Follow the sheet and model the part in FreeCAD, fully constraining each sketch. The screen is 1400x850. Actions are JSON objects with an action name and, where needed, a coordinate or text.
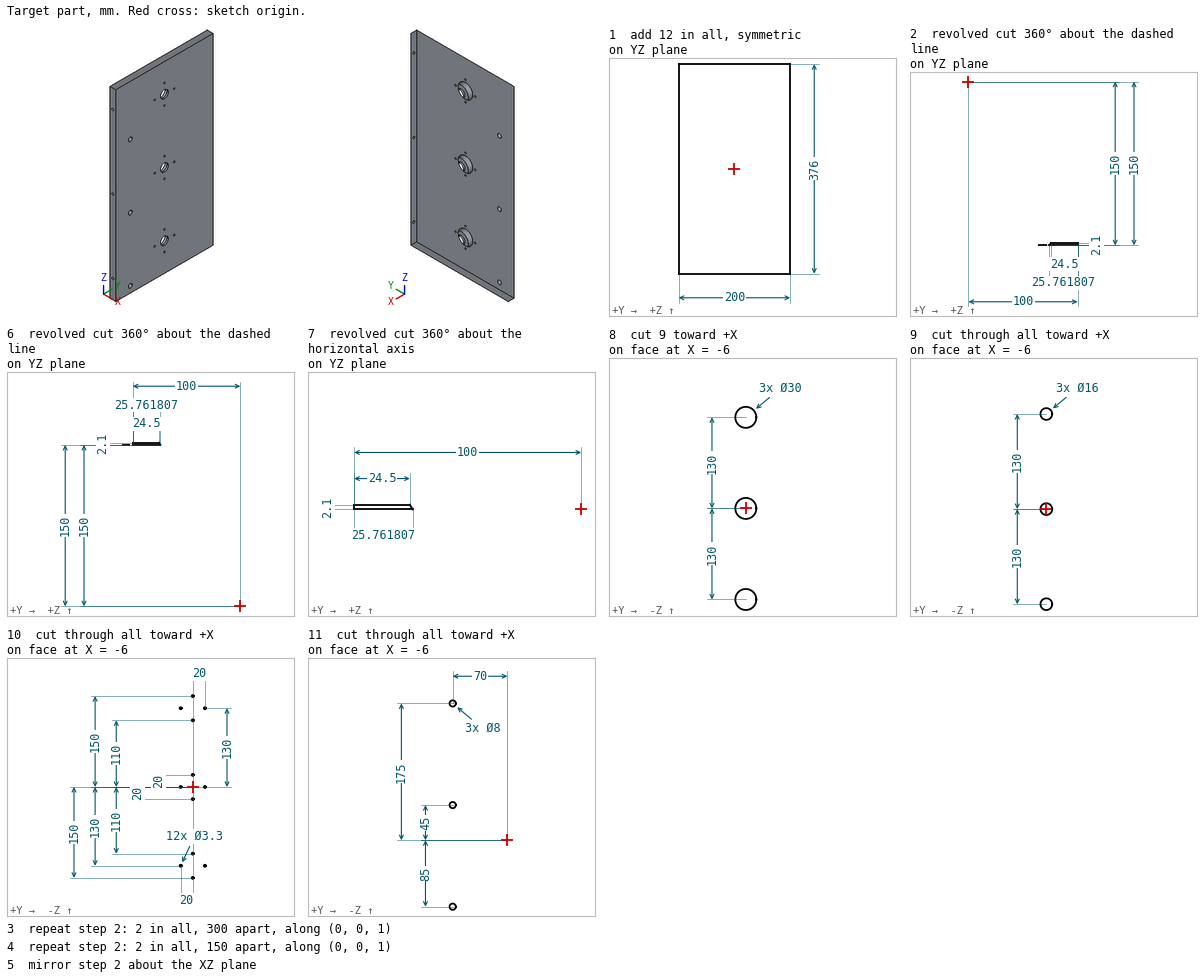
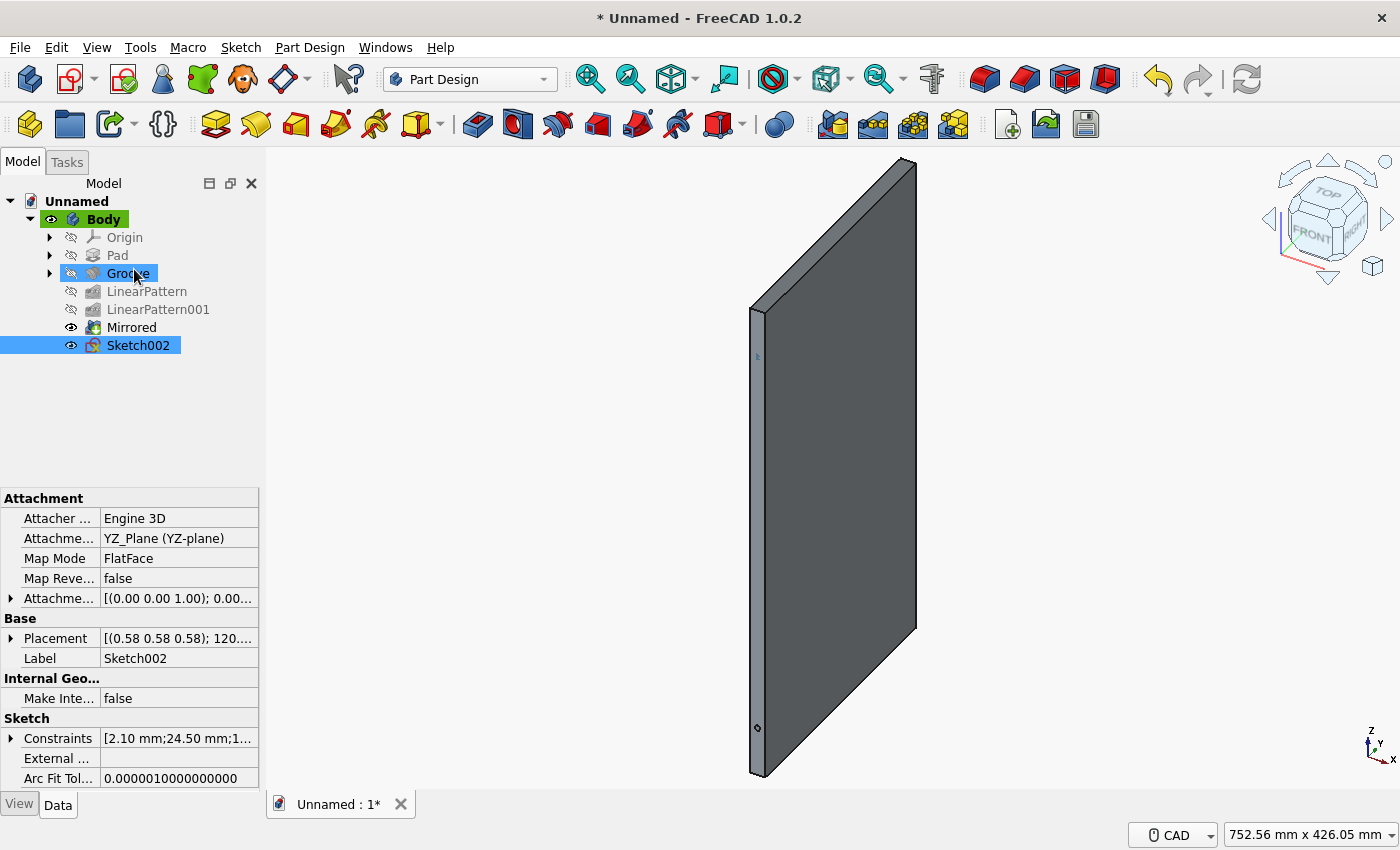
{"action": "left_click", "coordinate": [558, 124]}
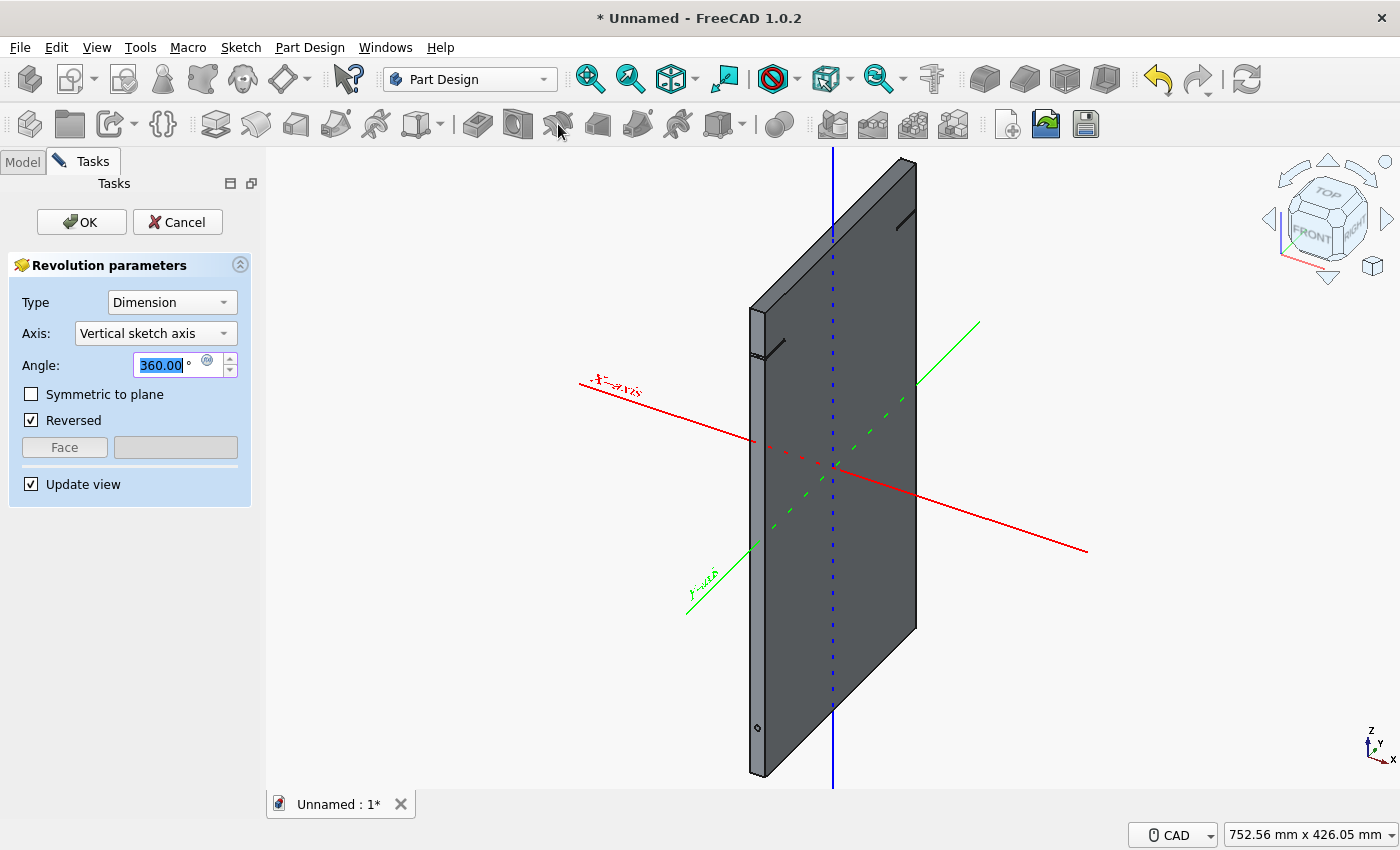
{"action": "left_click", "coordinate": [156, 334]}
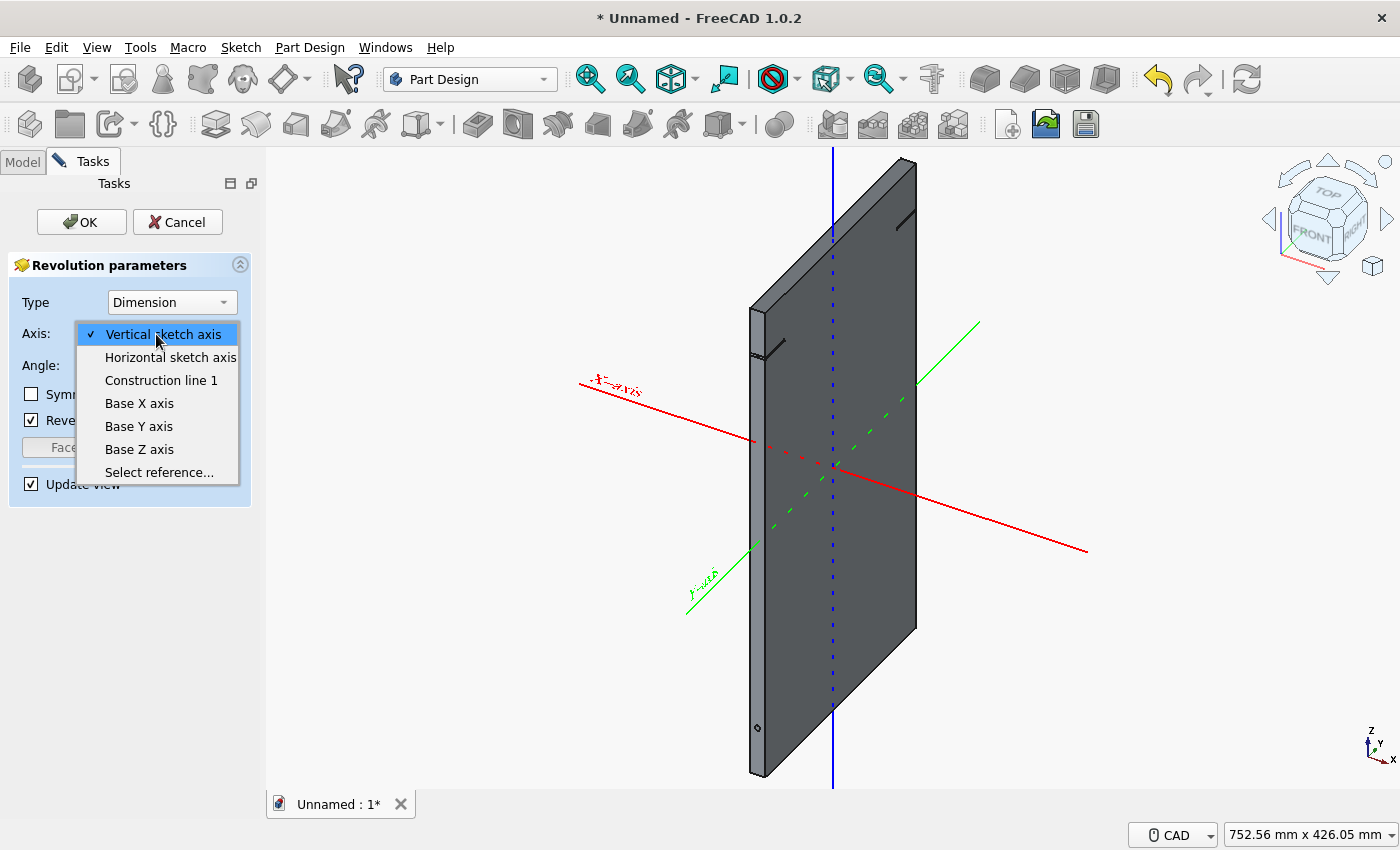
{"action": "left_click", "coordinate": [156, 380]}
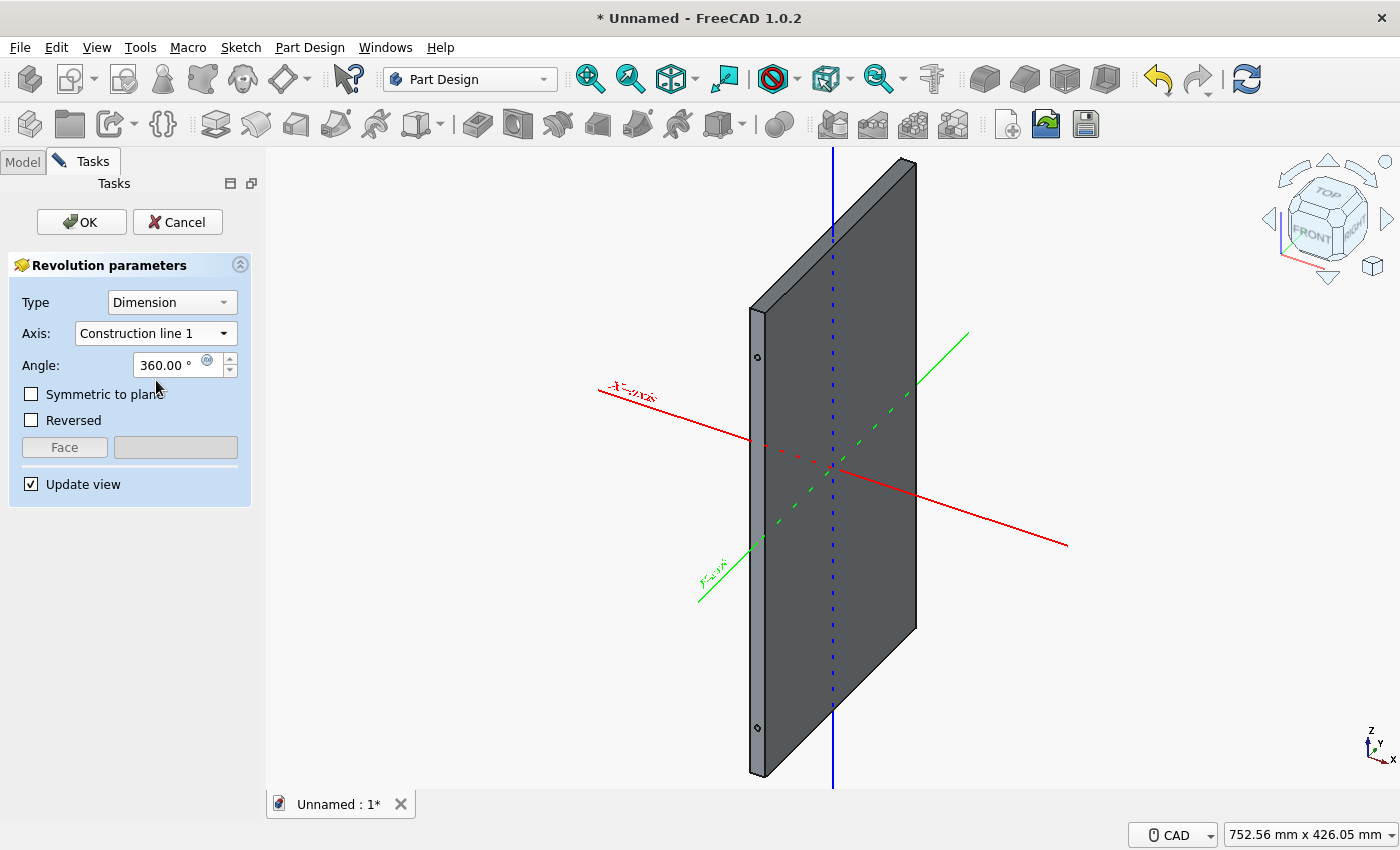
{"action": "left_click", "coordinate": [82, 222]}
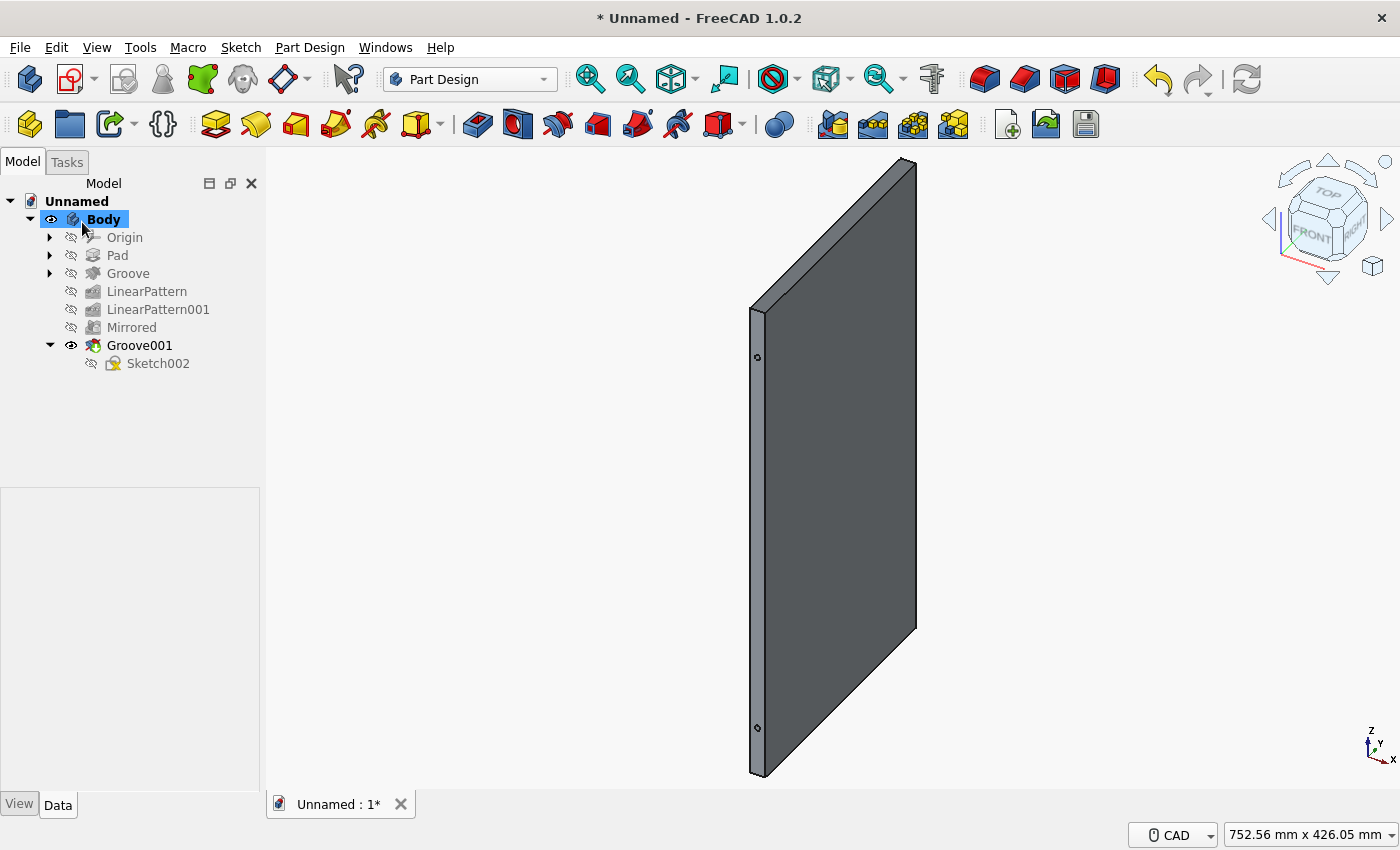
{"action": "left_click", "coordinate": [70, 80]}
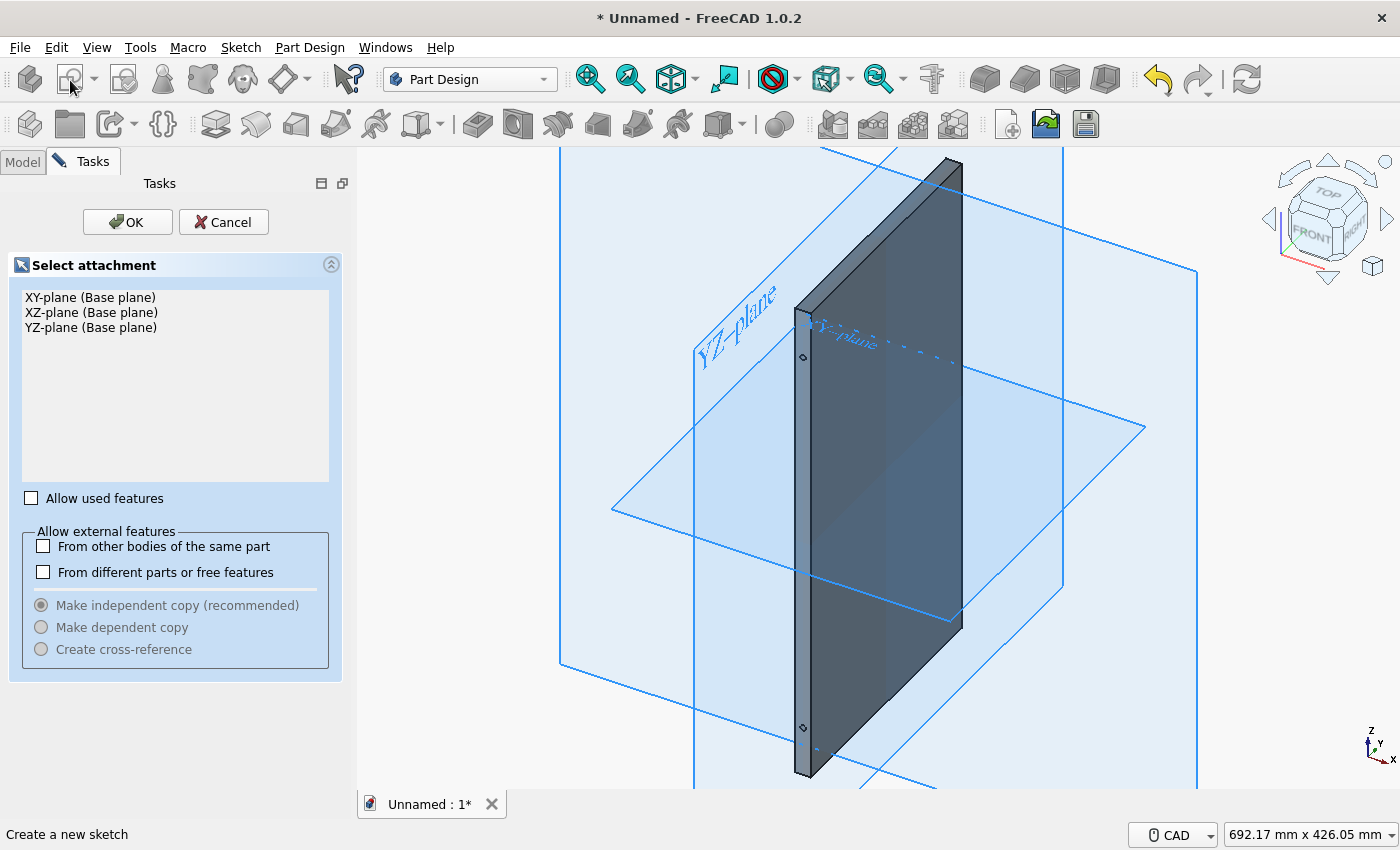
{"action": "left_click", "coordinate": [82, 328]}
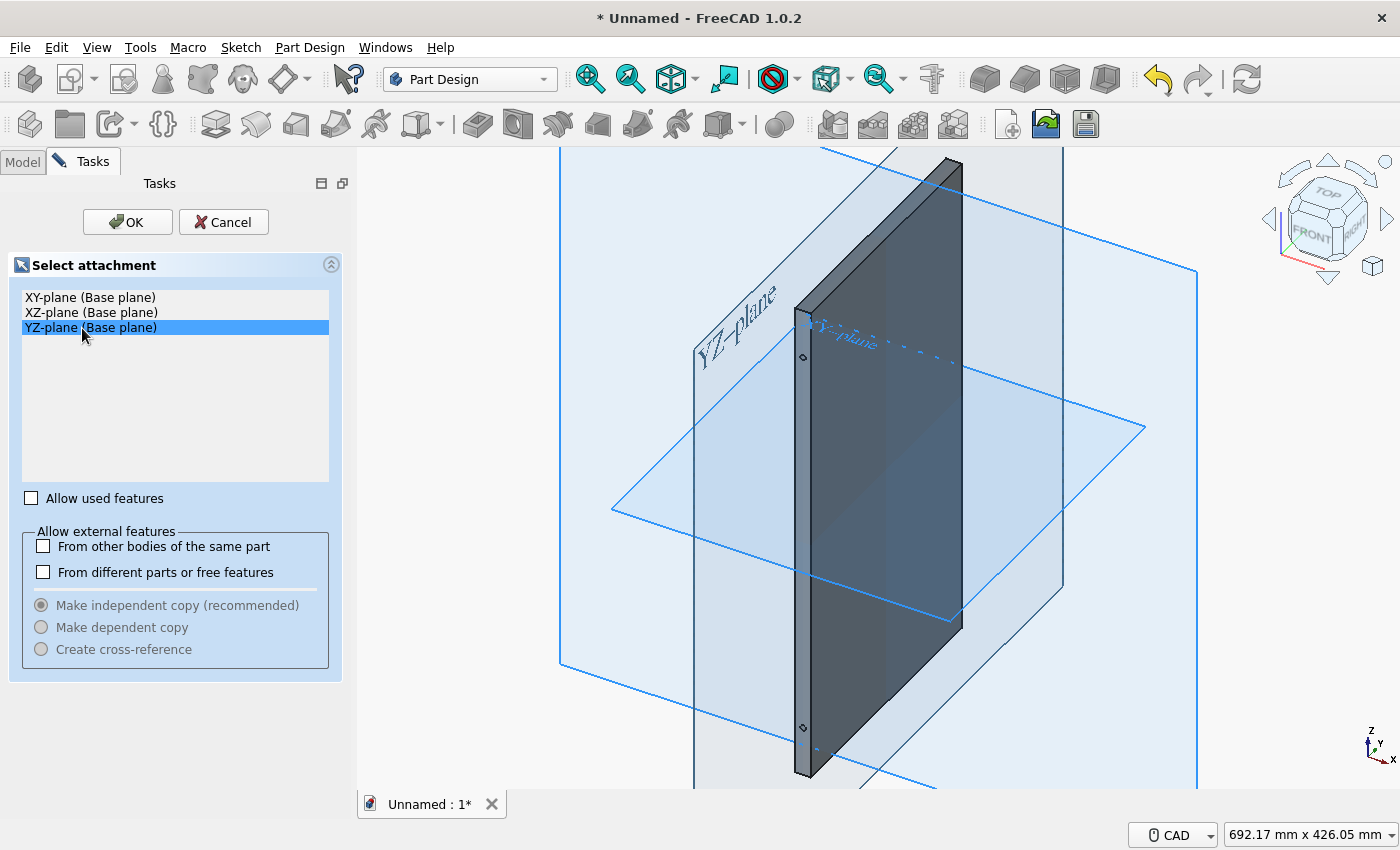
{"action": "left_click", "coordinate": [128, 222]}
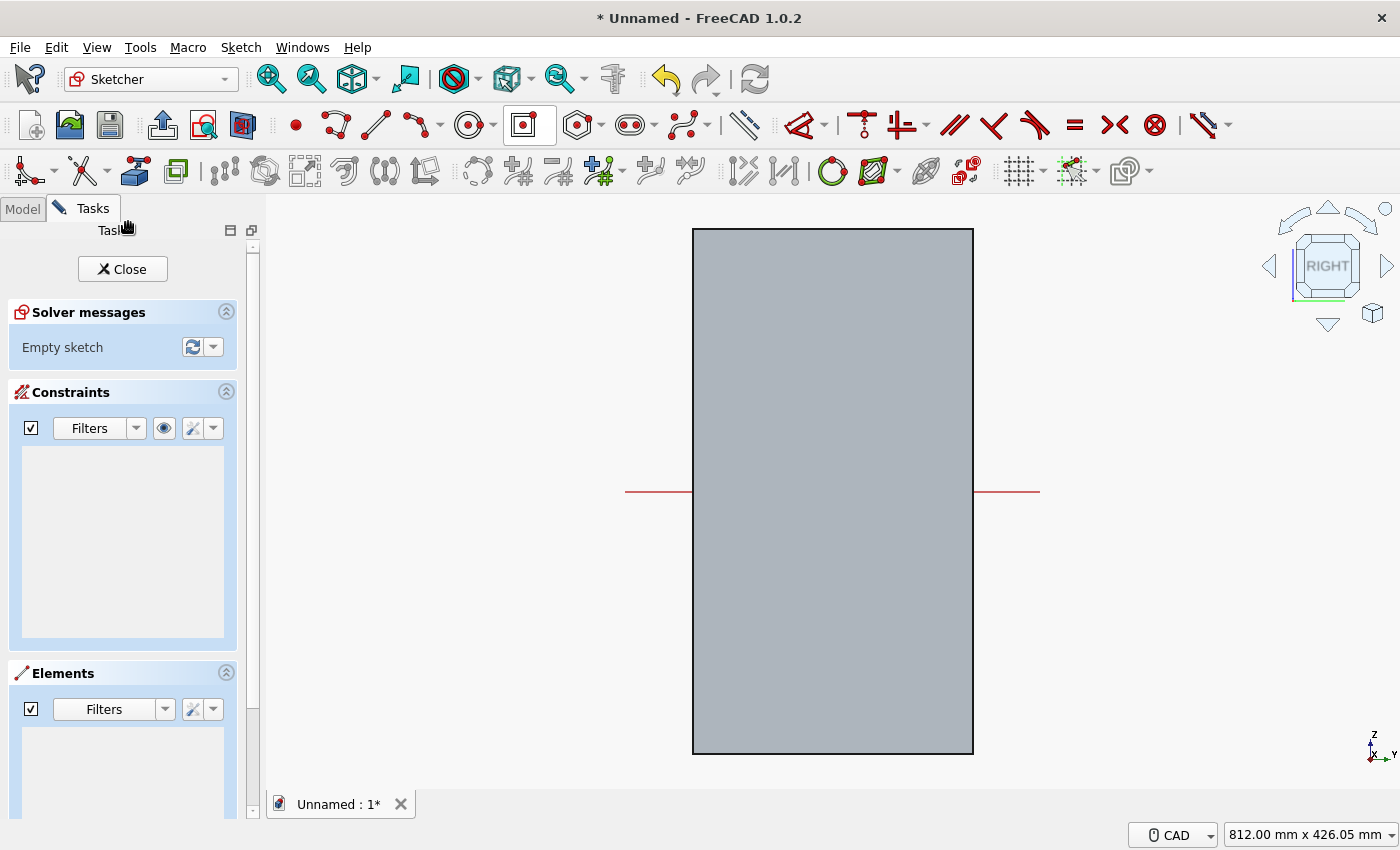
{"action": "left_click", "coordinate": [244, 126]}